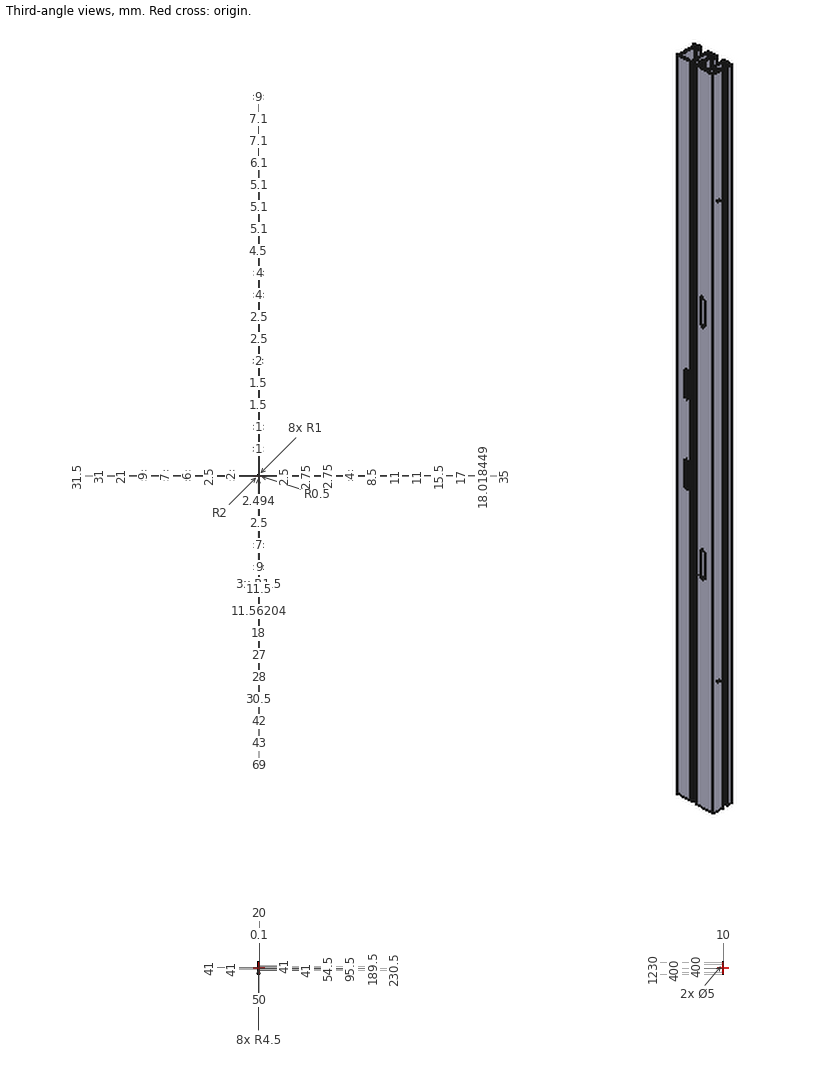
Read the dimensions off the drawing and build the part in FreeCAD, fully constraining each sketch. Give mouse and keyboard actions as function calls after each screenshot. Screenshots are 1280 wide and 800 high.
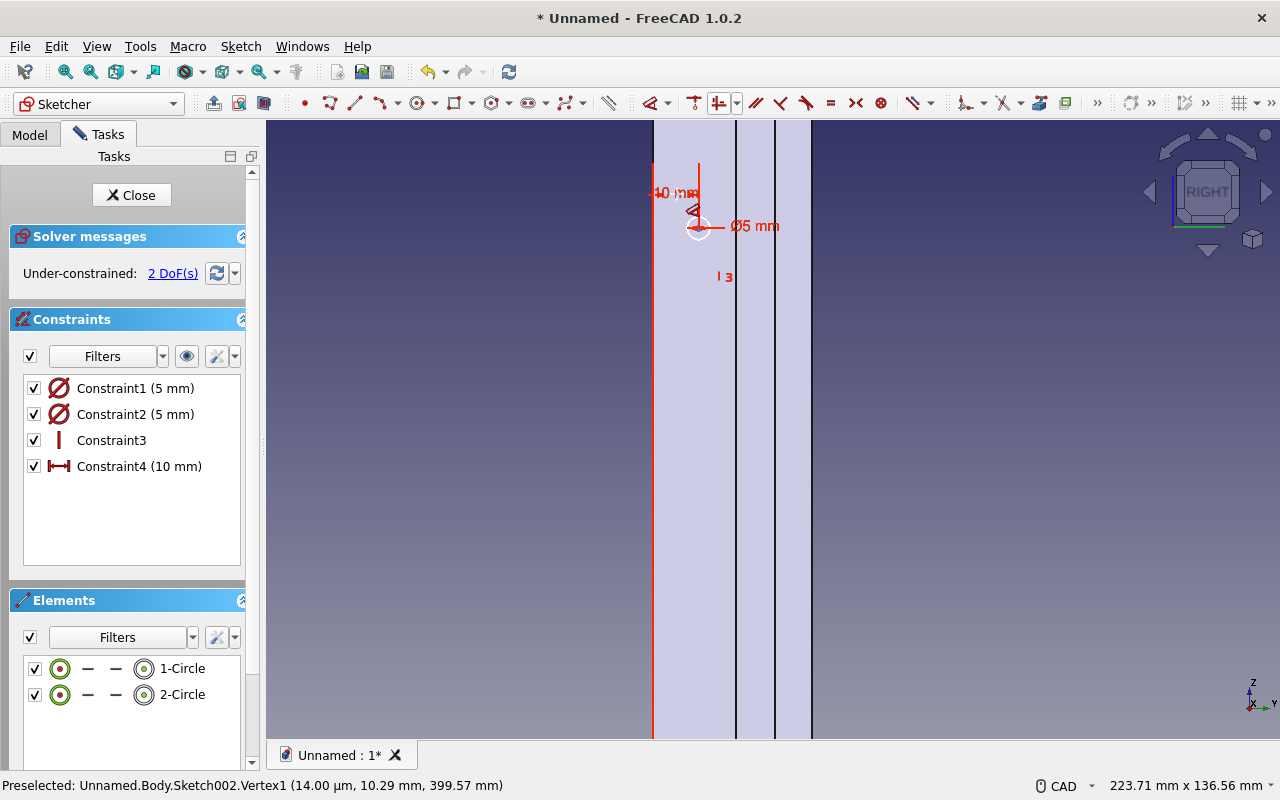
scroll(707, 229, down, 11)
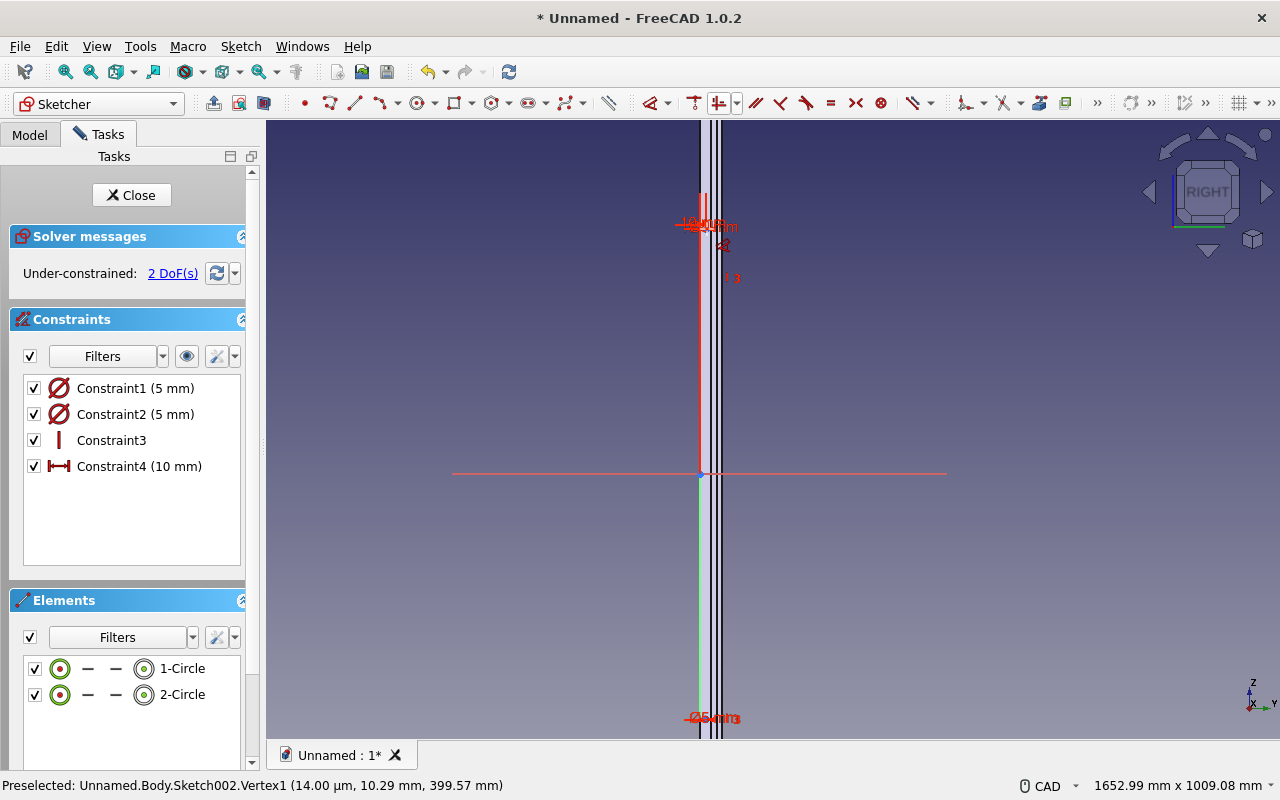
click(706, 229)
click(667, 329)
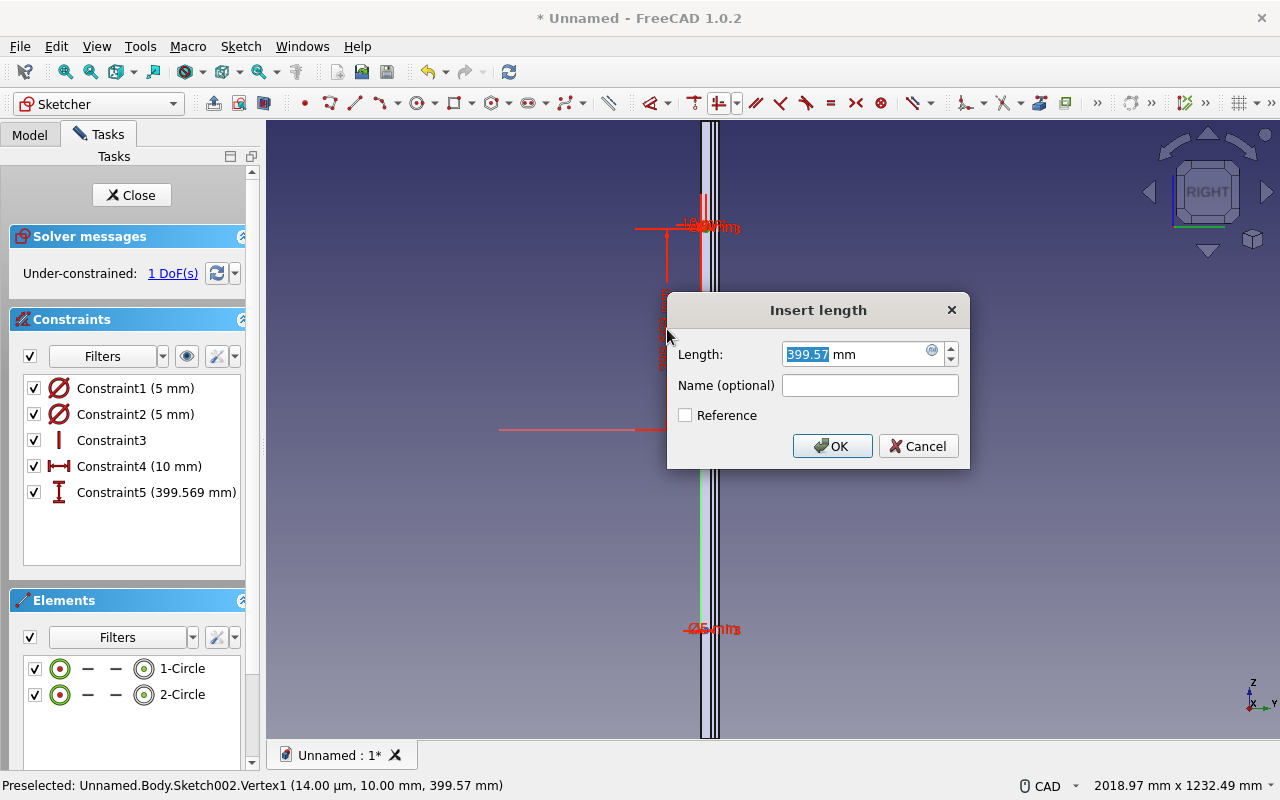
text(400)
key(Return)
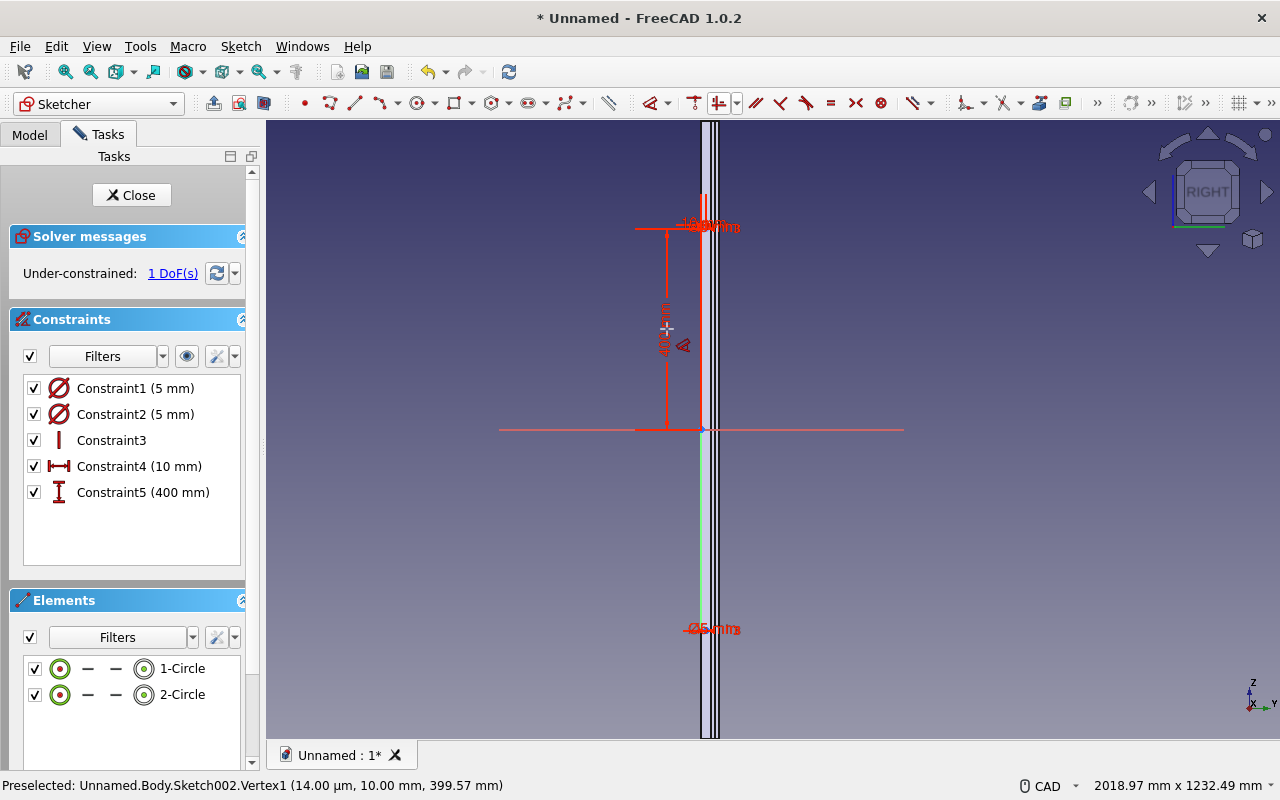
click(706, 631)
click(667, 530)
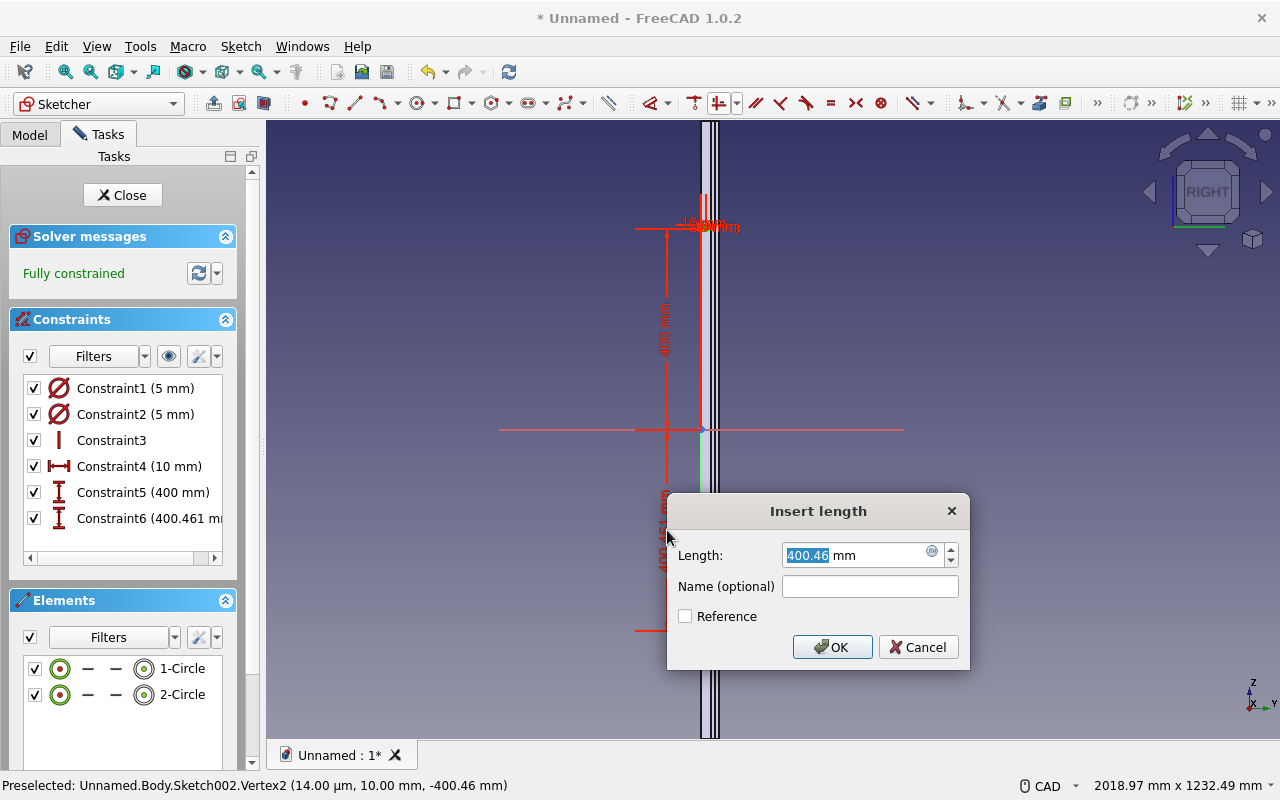
text(400)
key(Return)
key(Escape)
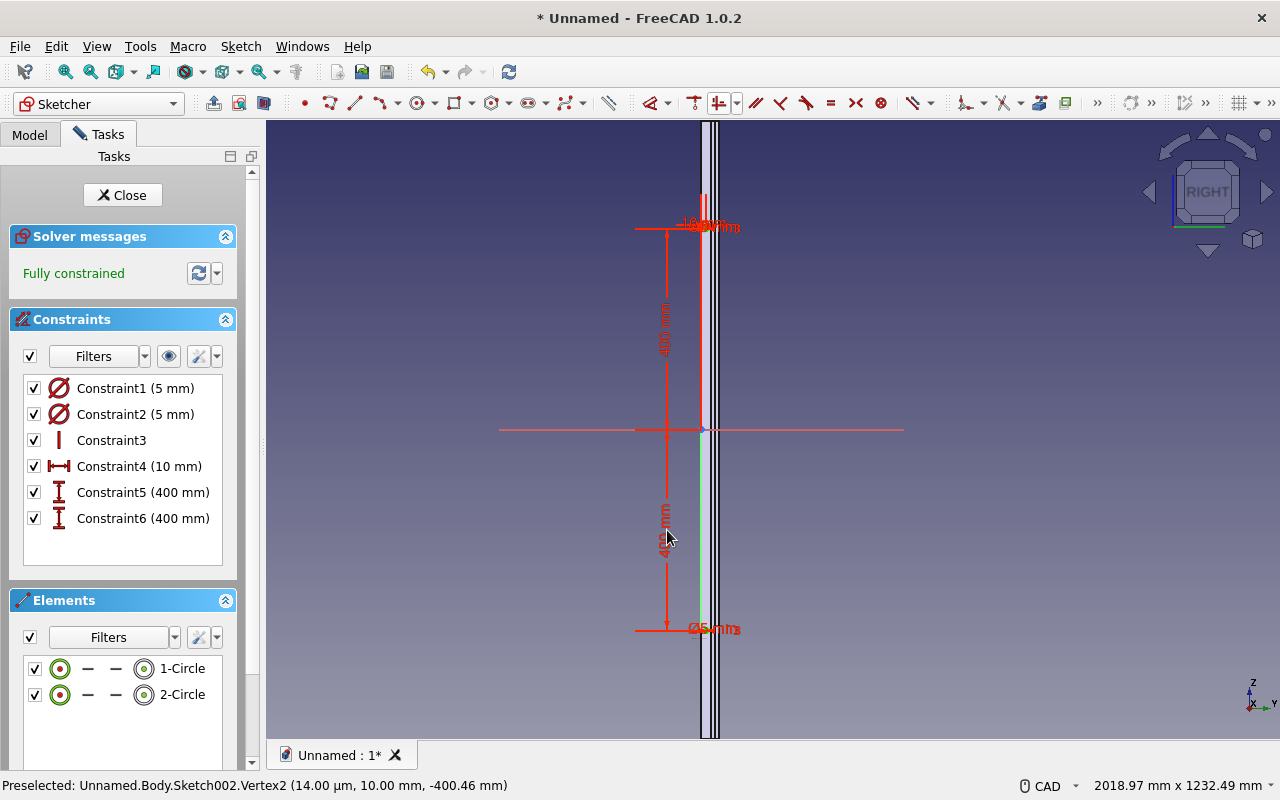
click(123, 195)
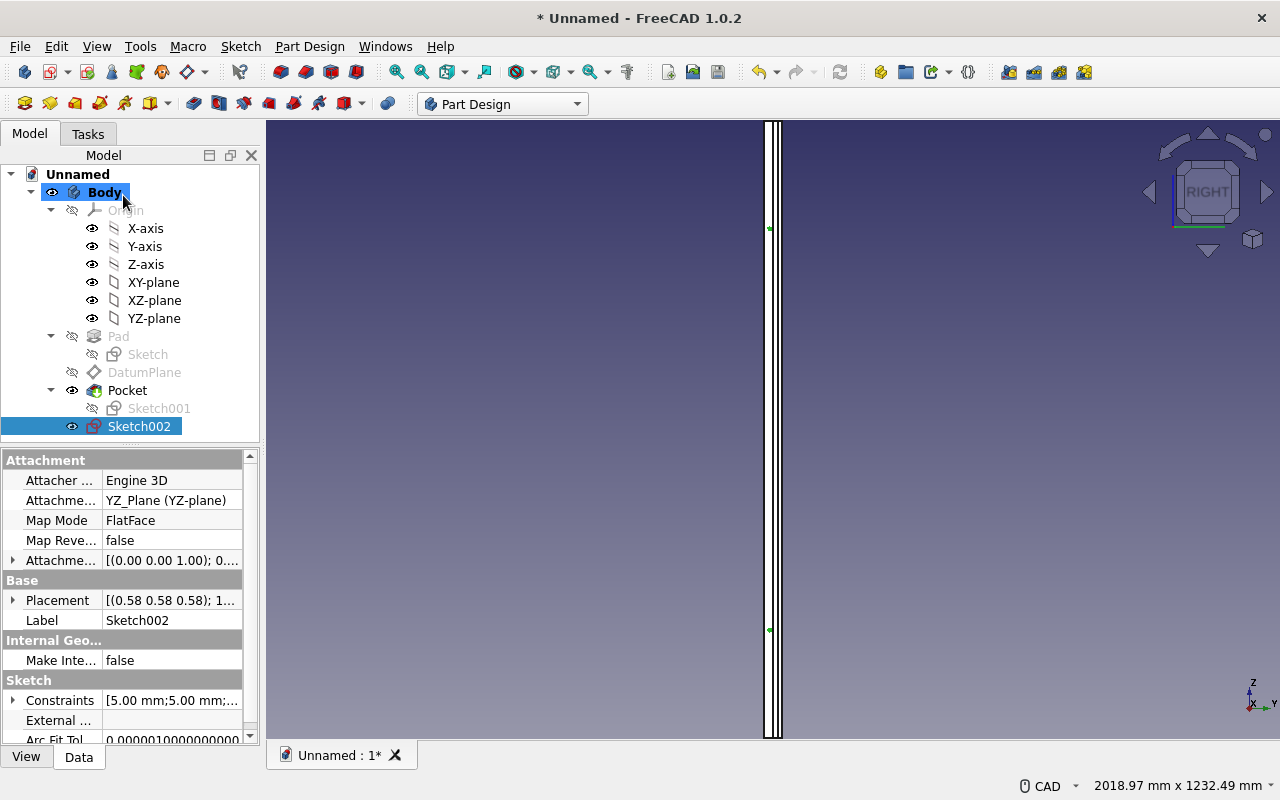
click(194, 104)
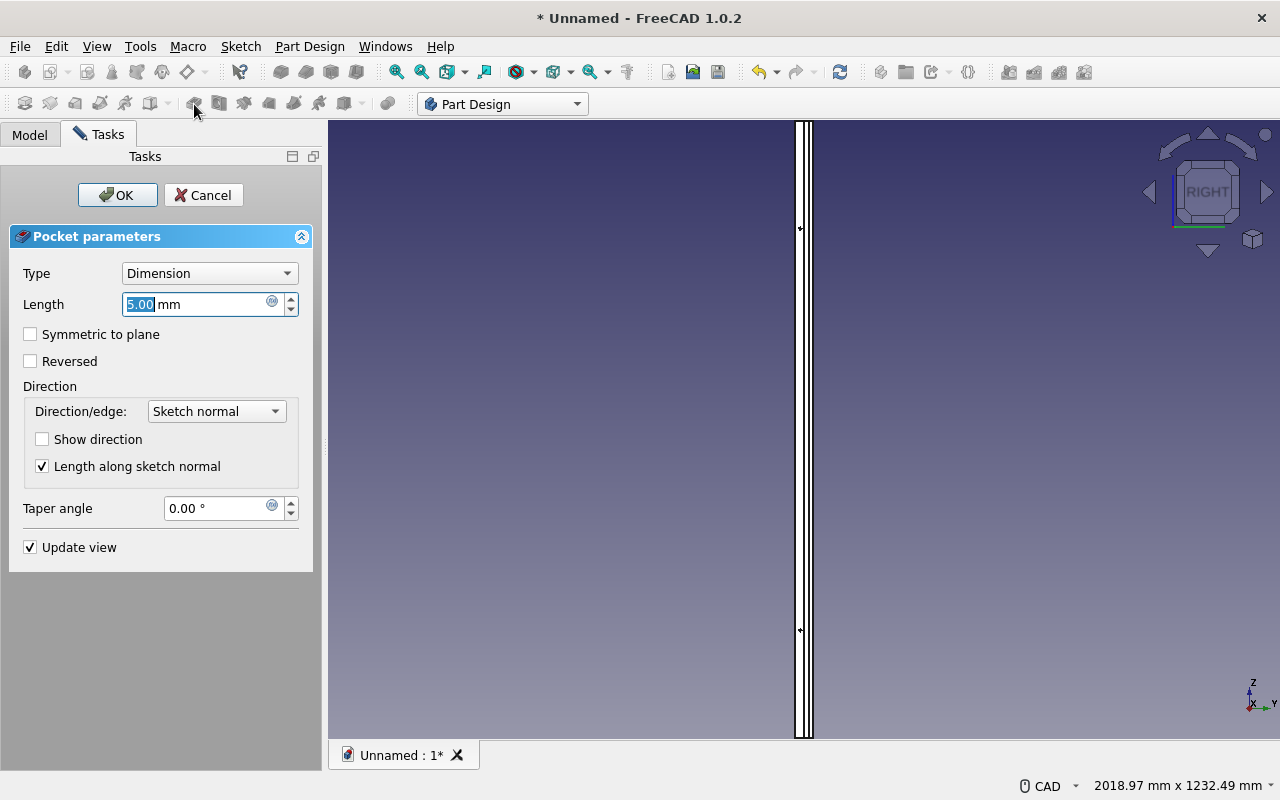
text(0.1)
key(Tab)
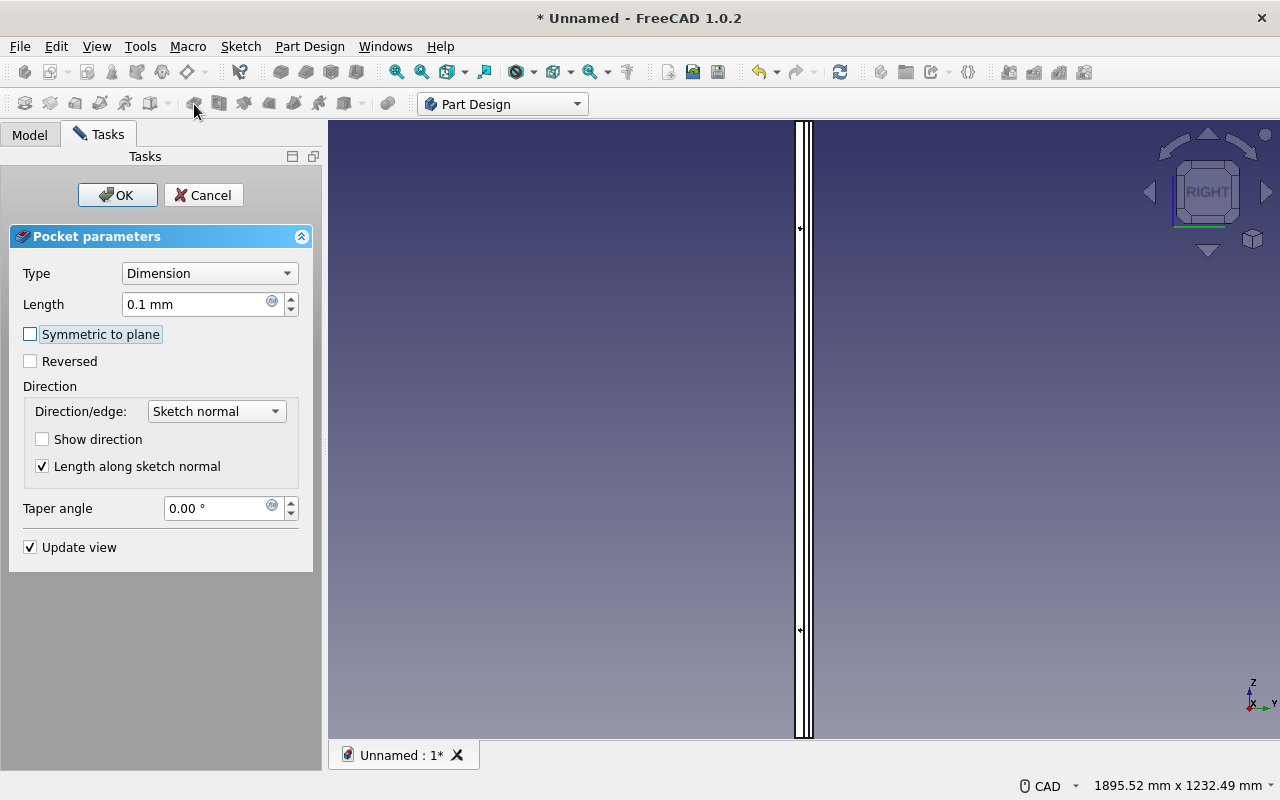
click(118, 195)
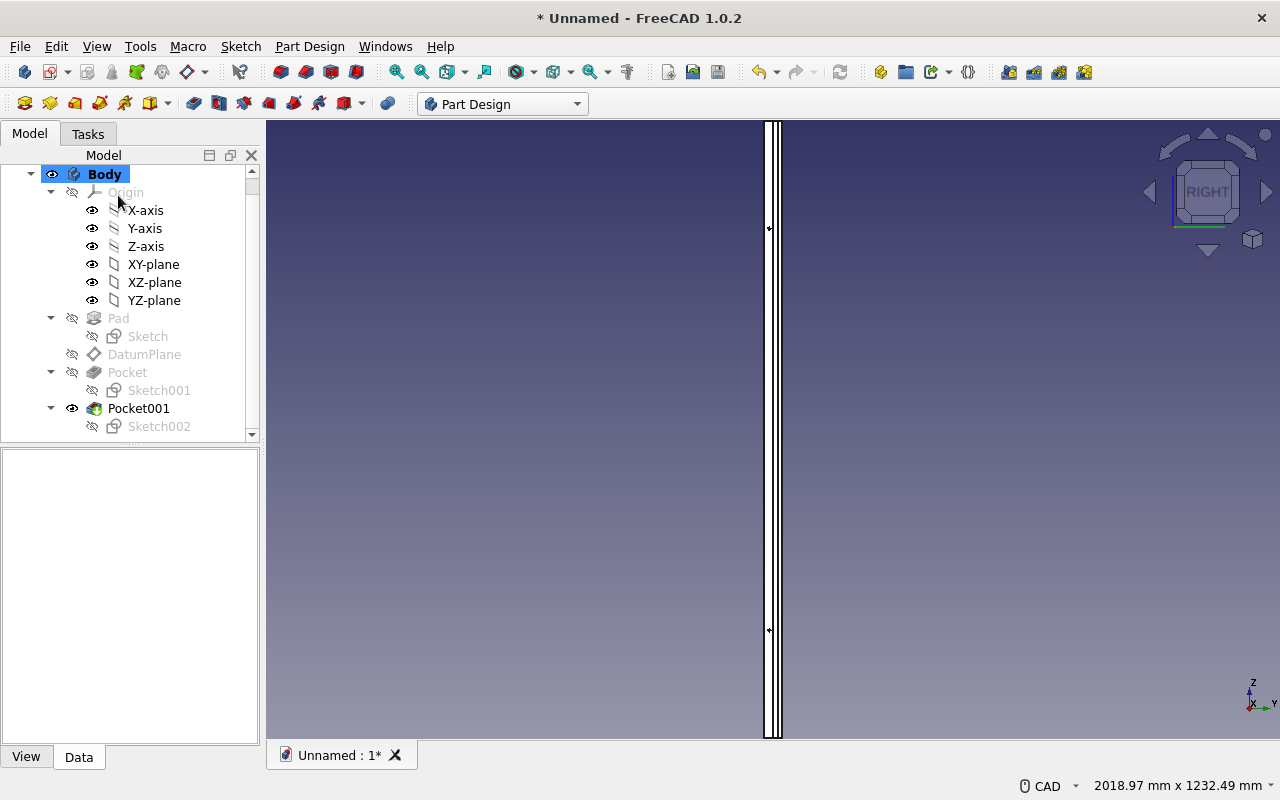
key(0)